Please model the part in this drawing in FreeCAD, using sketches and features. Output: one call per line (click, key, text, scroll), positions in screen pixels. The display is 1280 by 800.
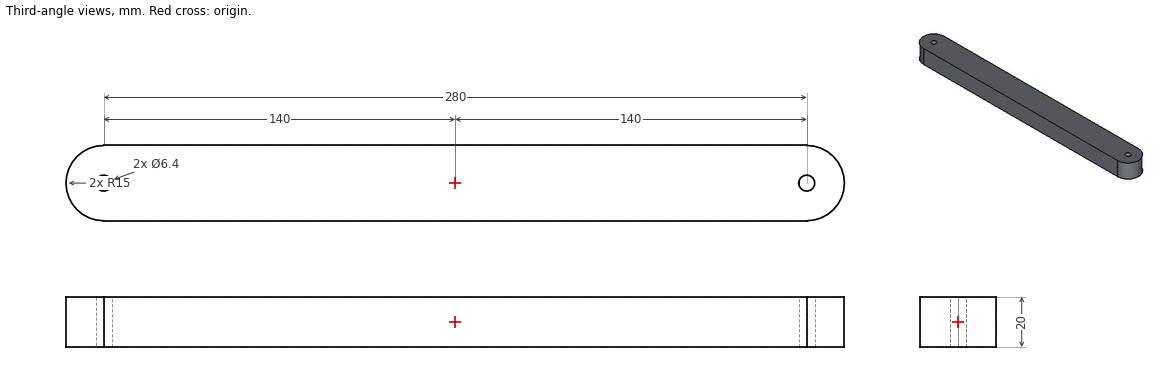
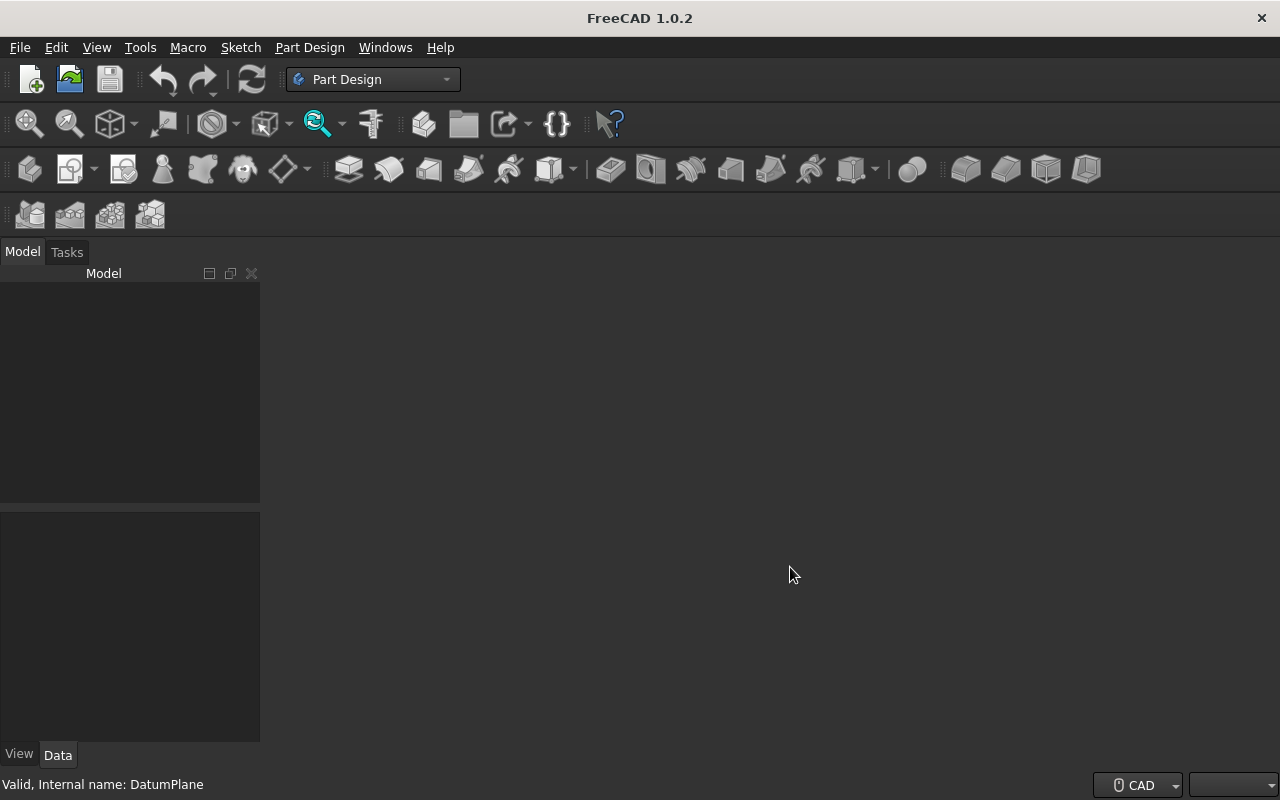
click(30, 80)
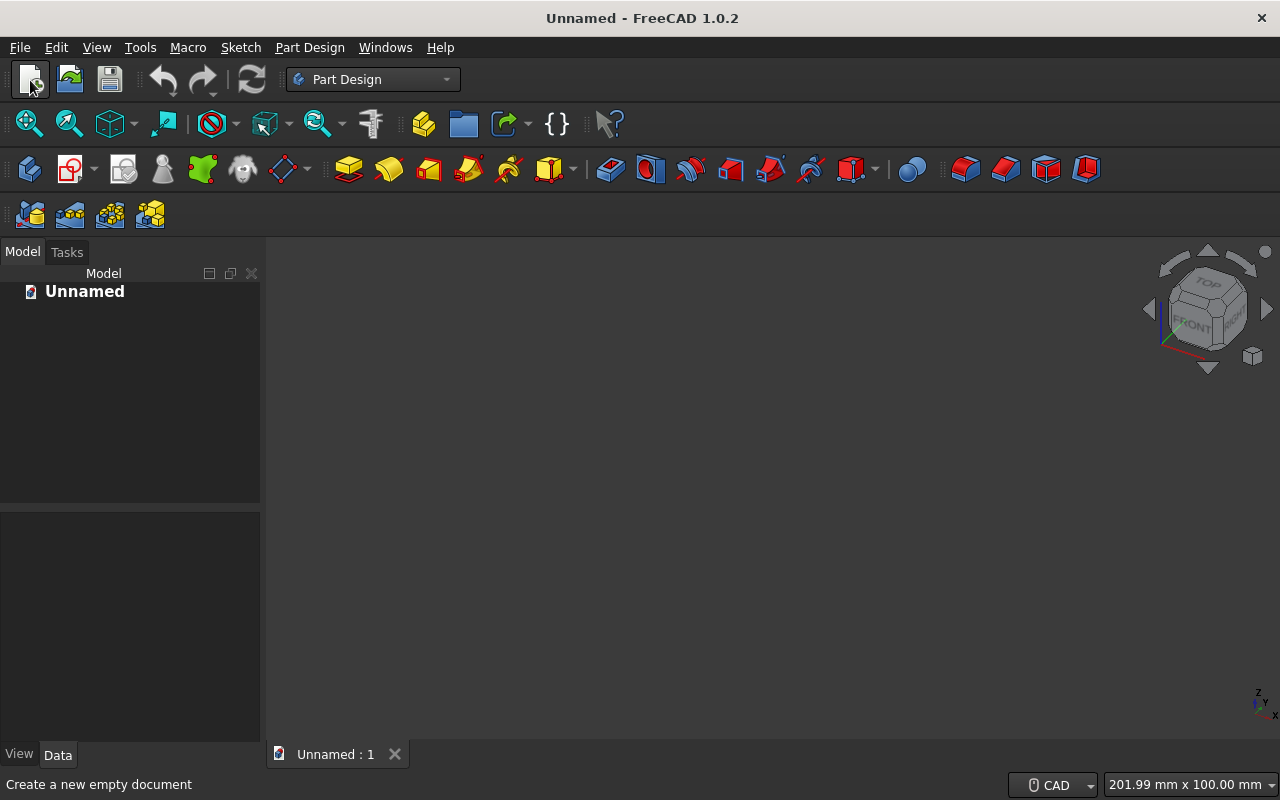
click(70, 170)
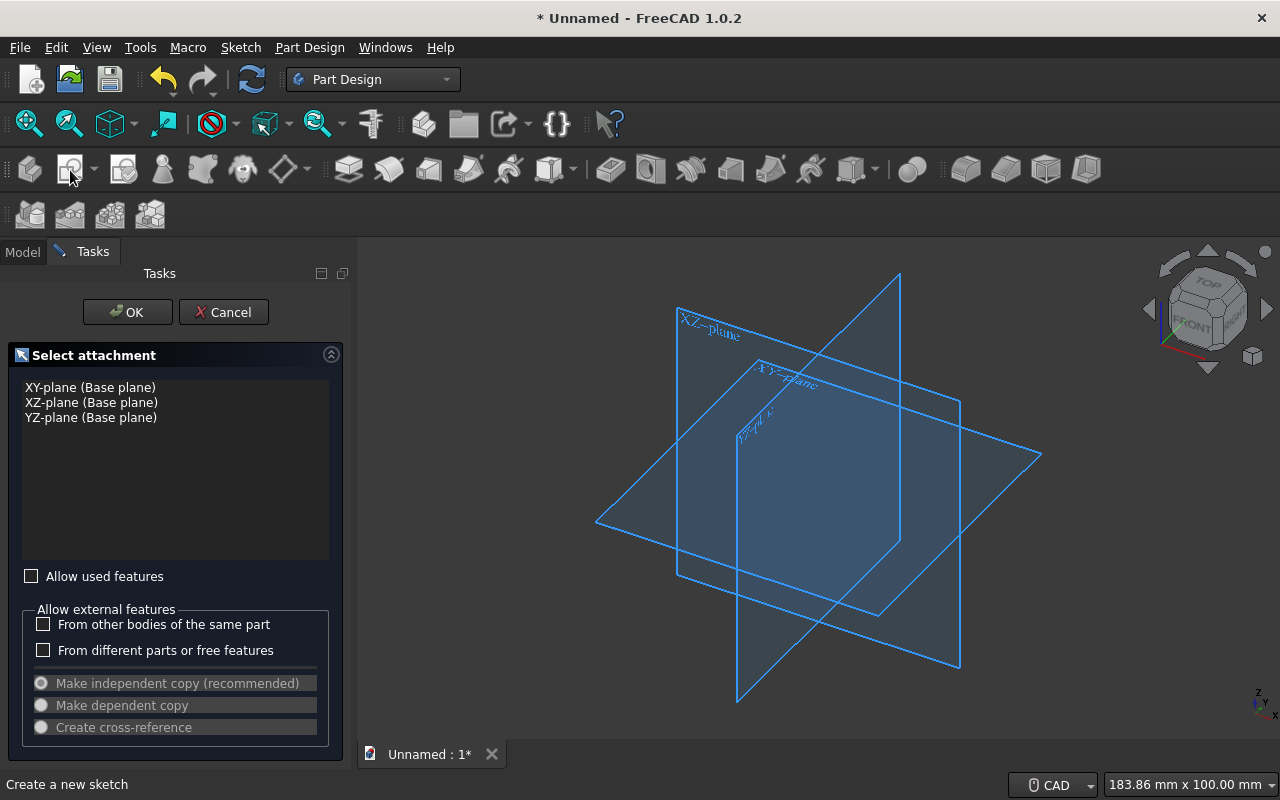
click(82, 388)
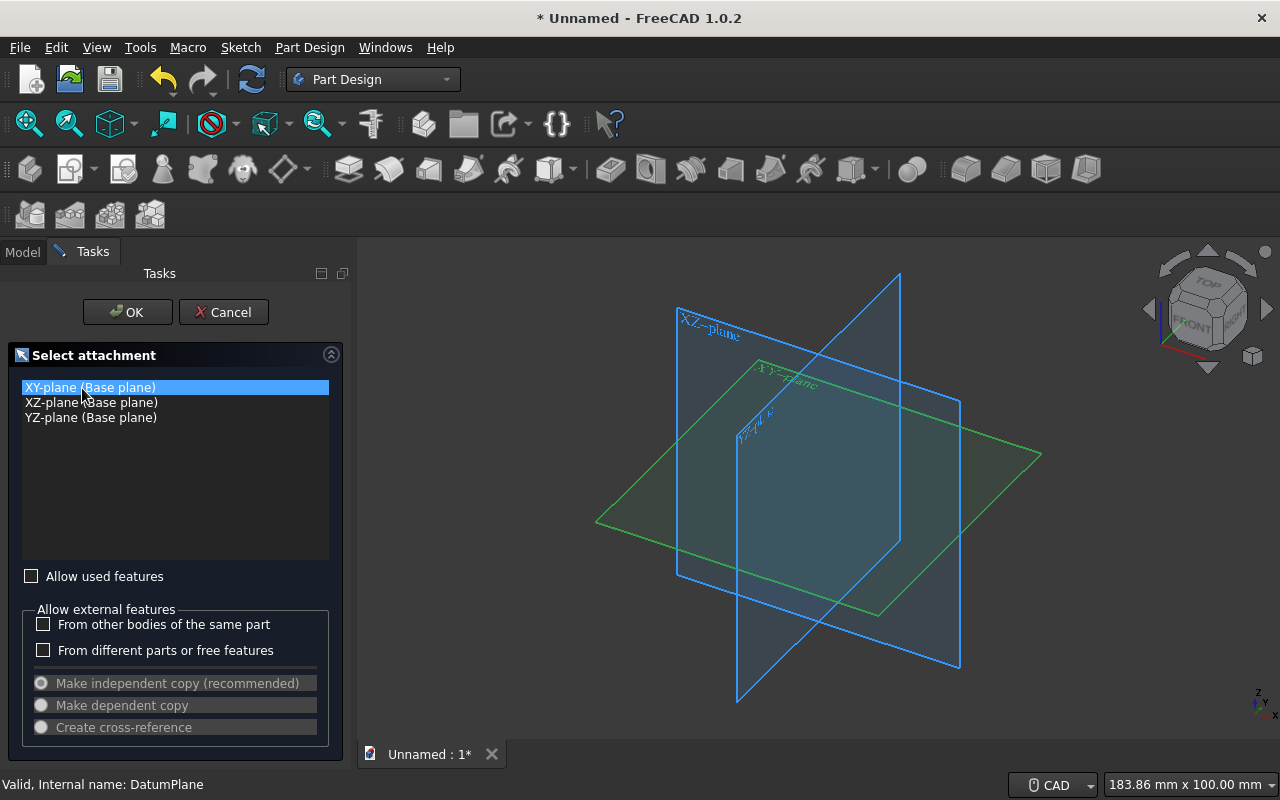
click(128, 312)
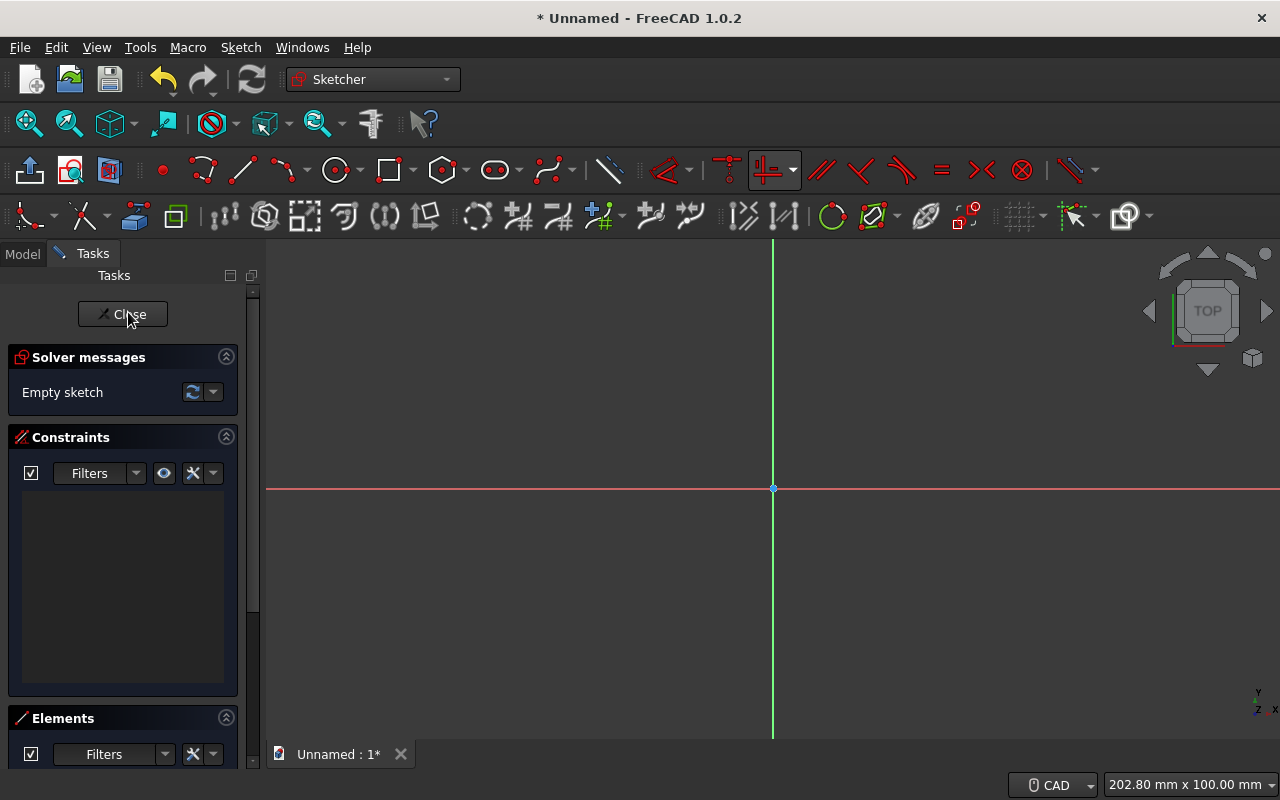
scroll(665, 489, down, 5)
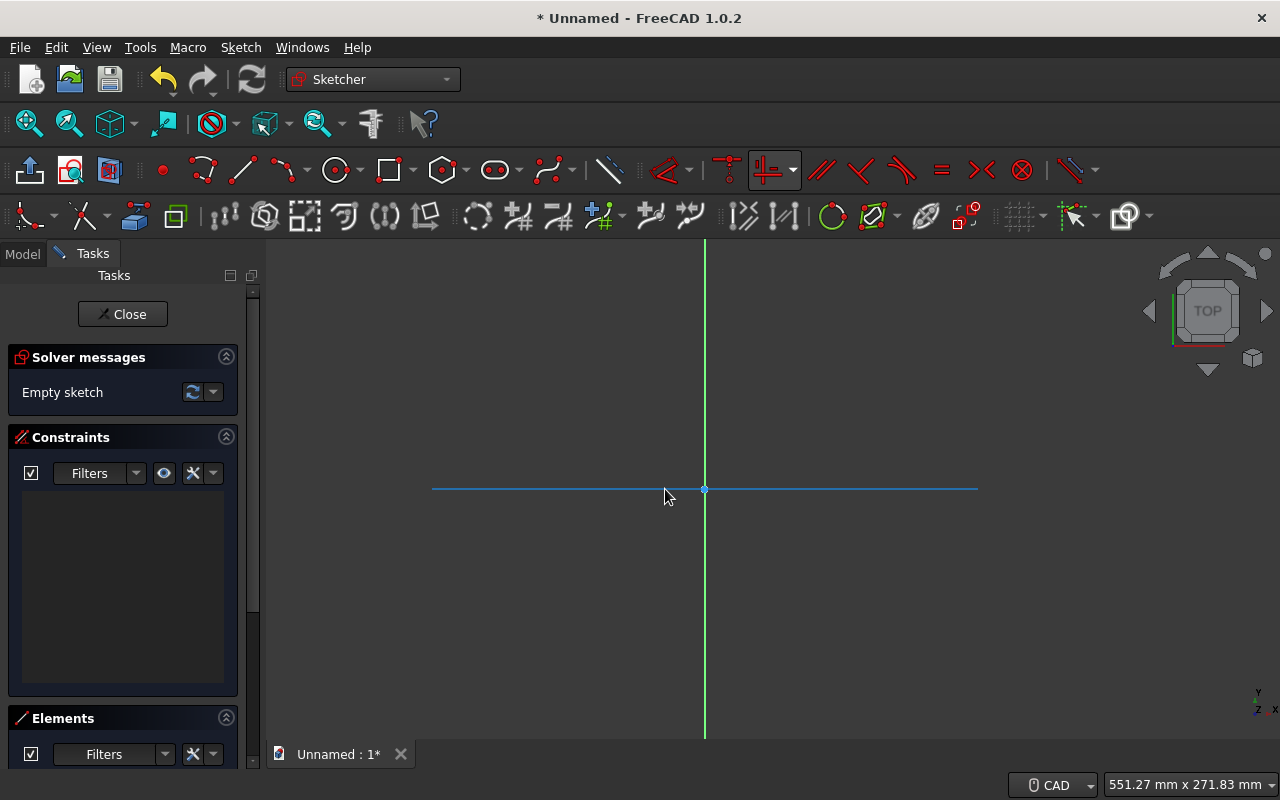
click(496, 170)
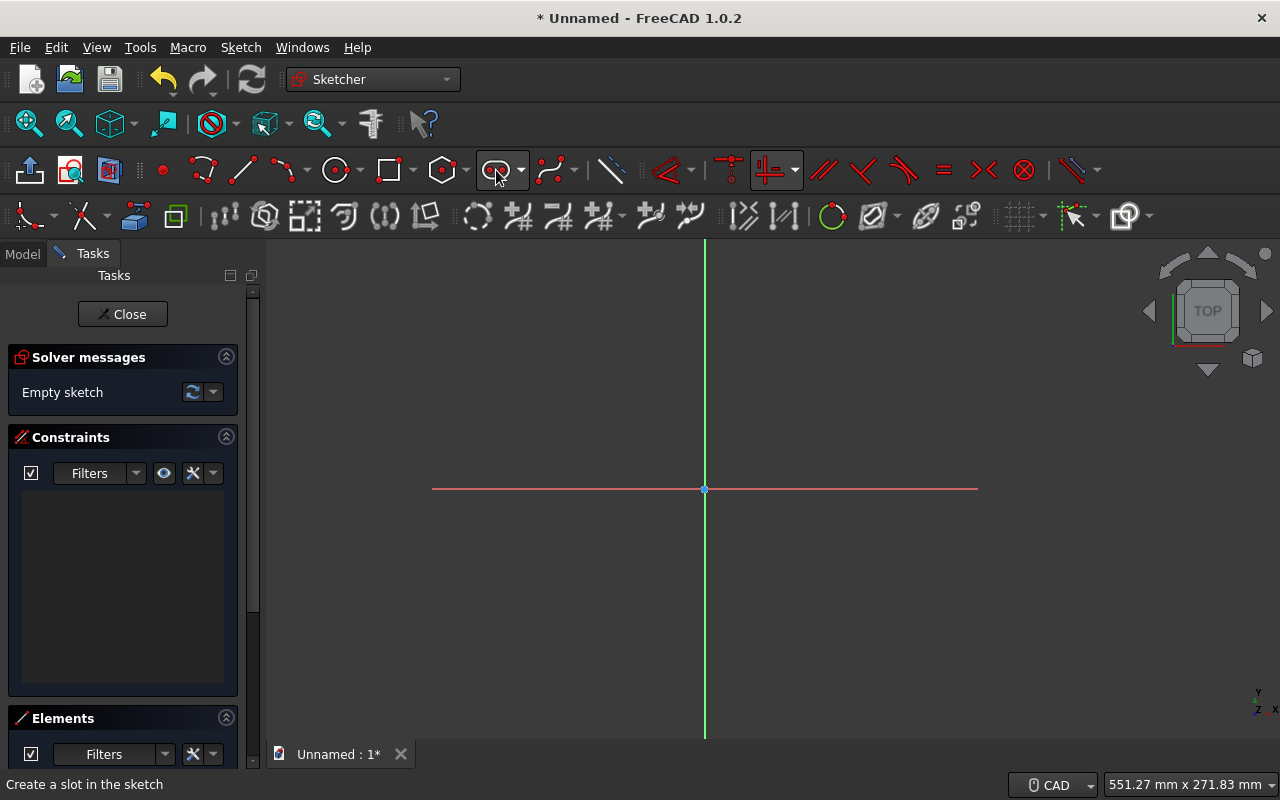
click(447, 489)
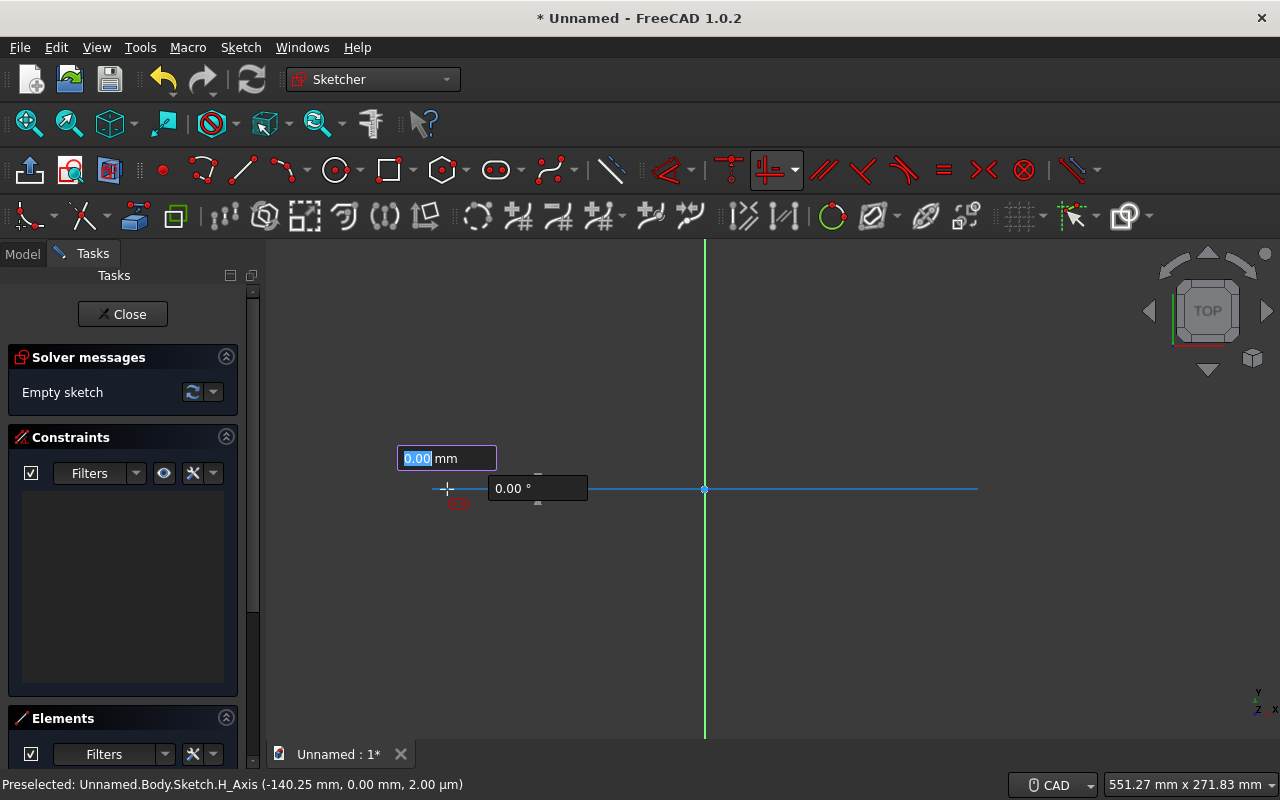
click(962, 480)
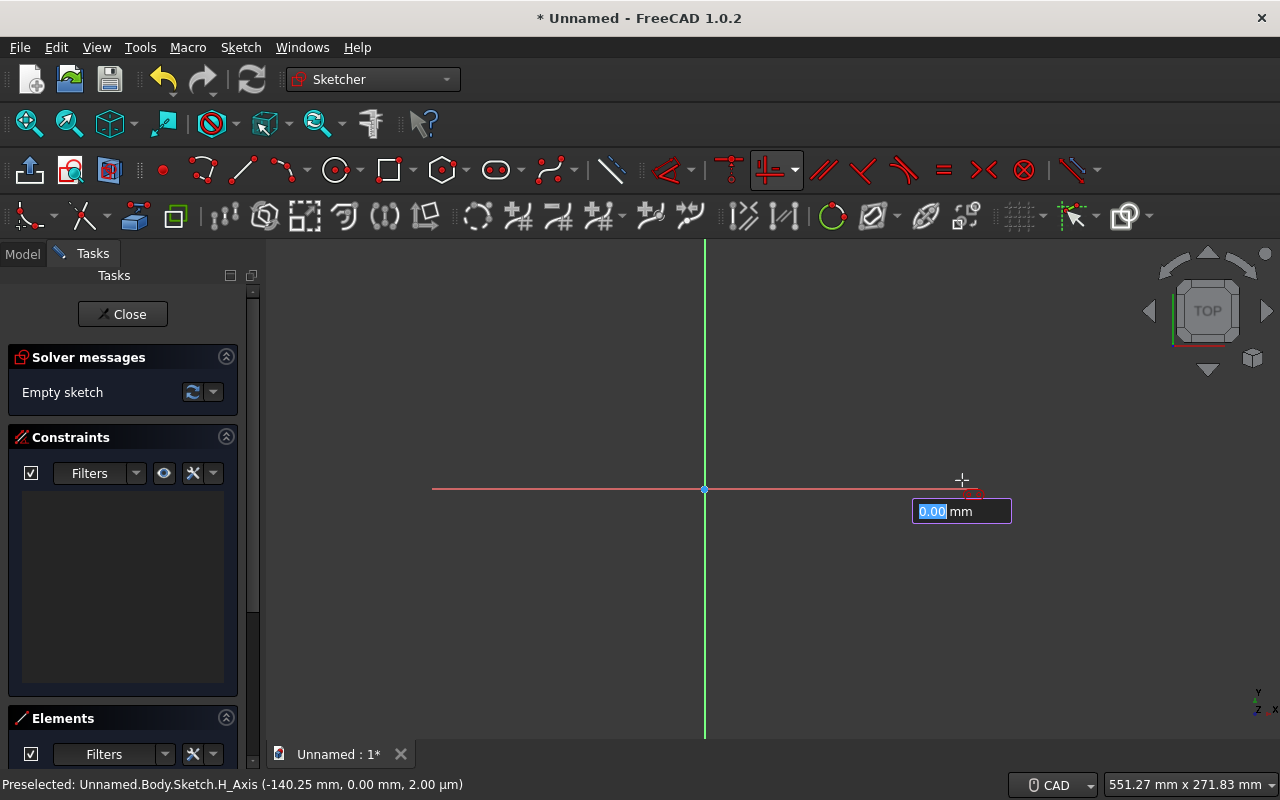
click(782, 462)
key(Escape)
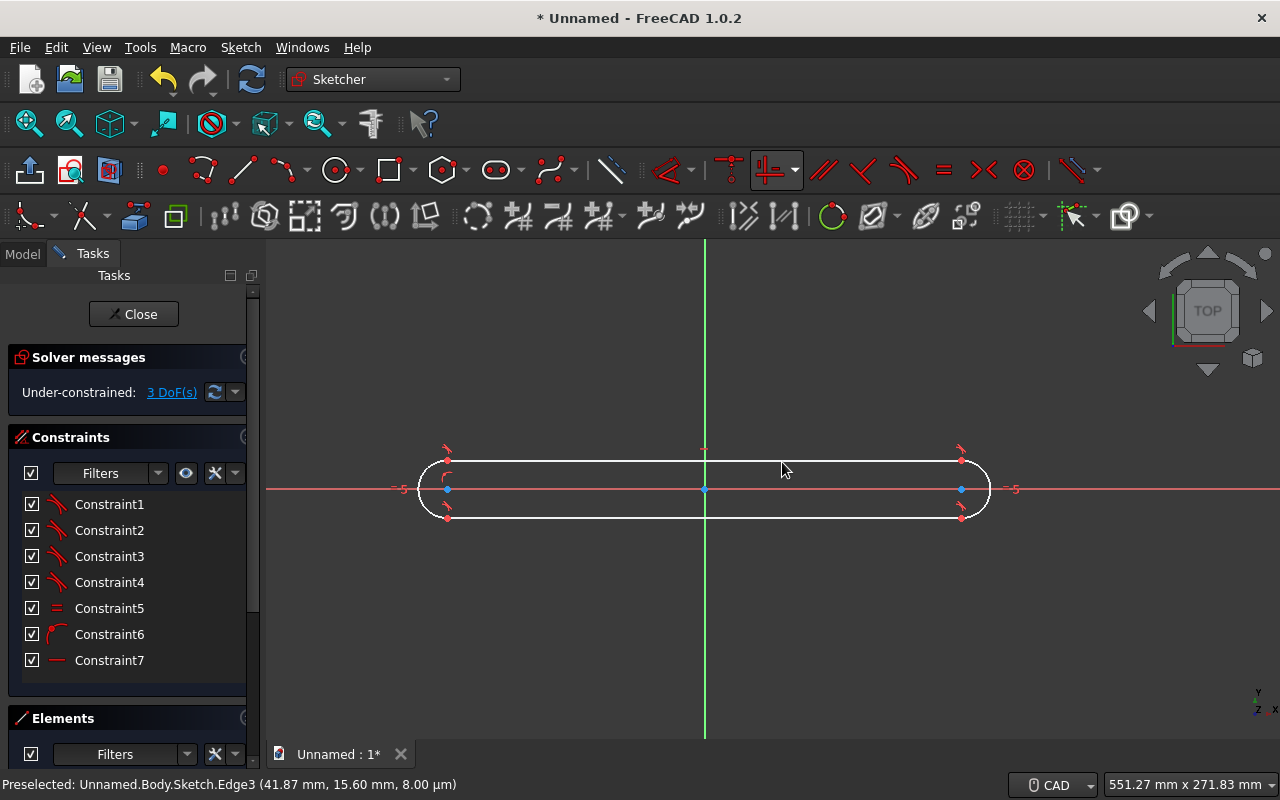
scroll(424, 472, up, 2)